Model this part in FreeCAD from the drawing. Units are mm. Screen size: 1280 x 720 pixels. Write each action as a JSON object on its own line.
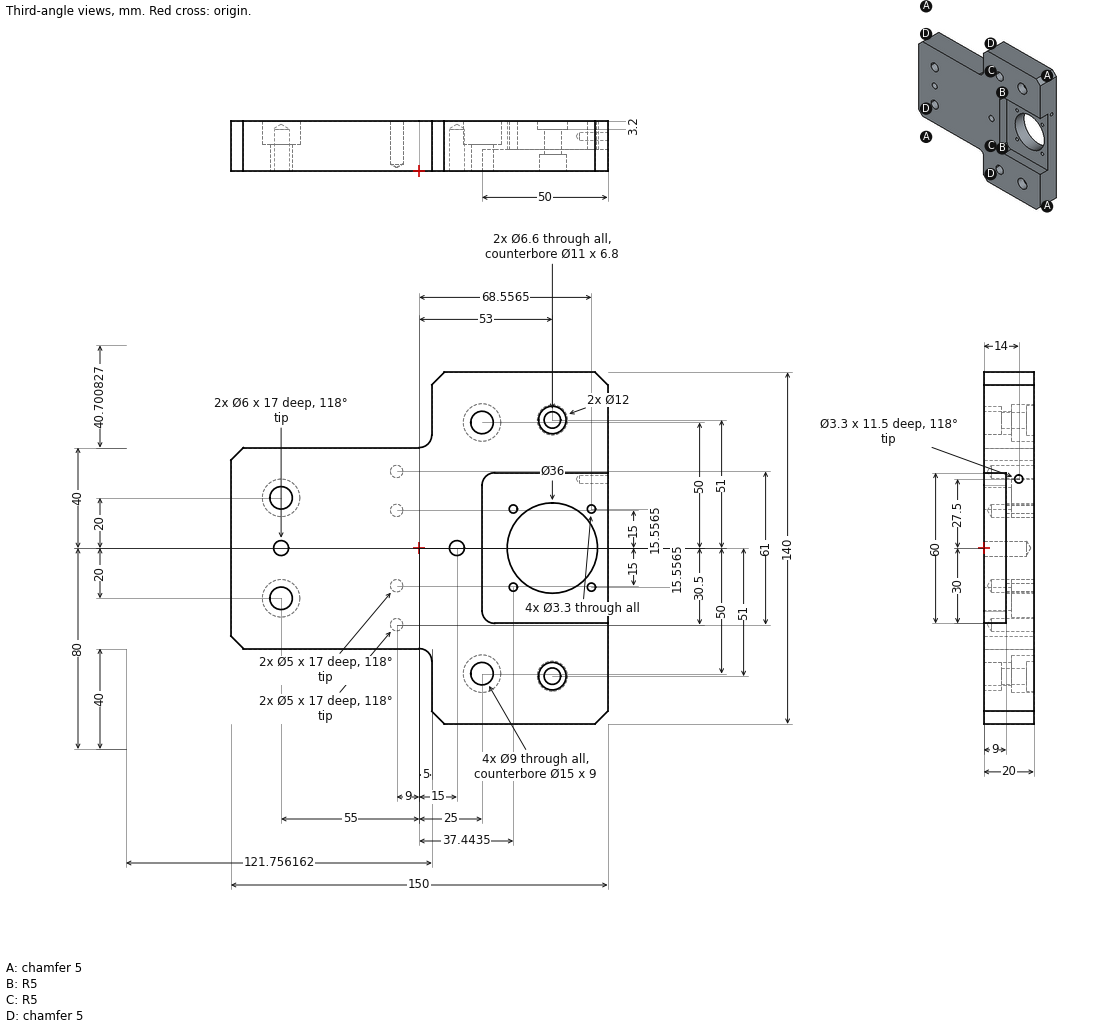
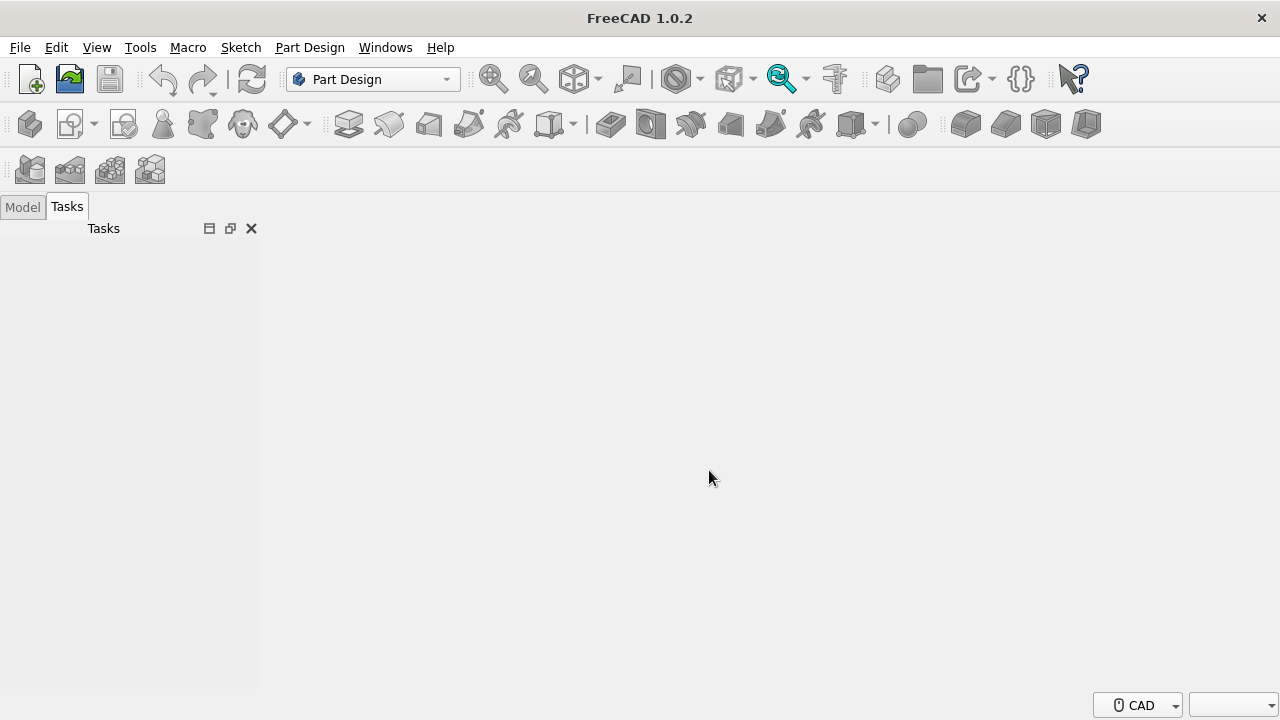
{"action": "left_click", "coordinate": [30, 80]}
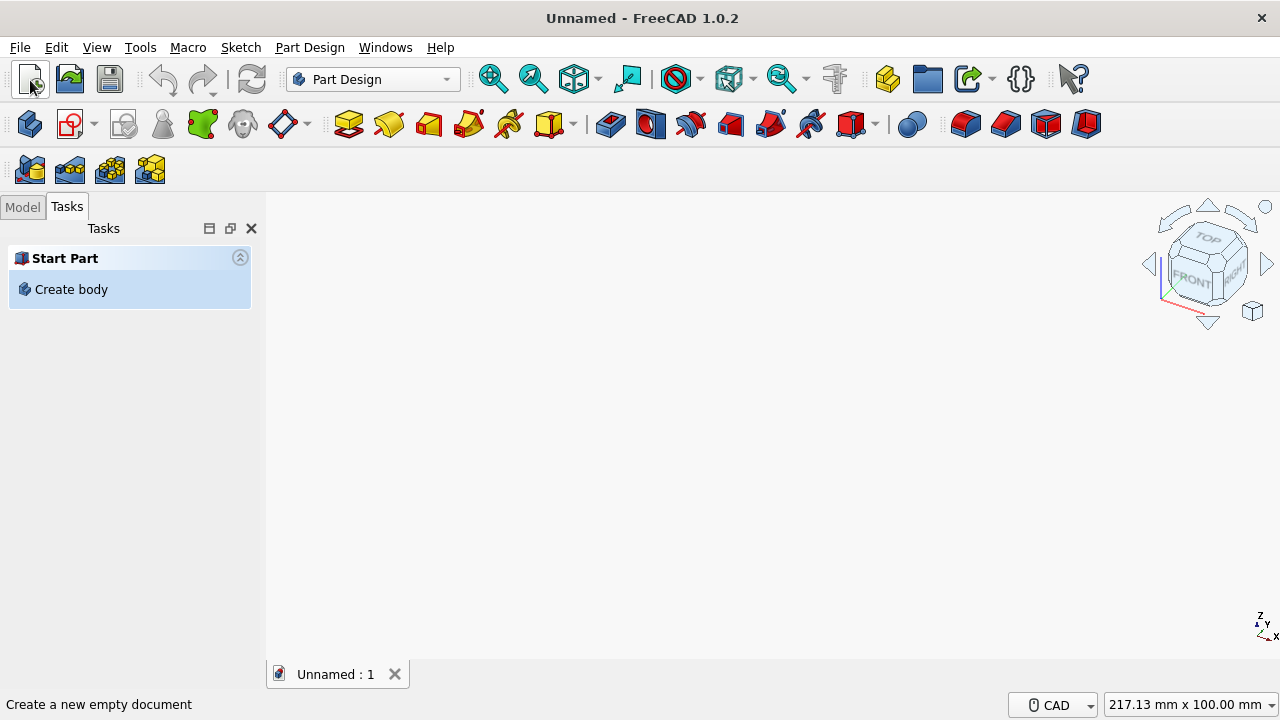
{"action": "left_click", "coordinate": [70, 124]}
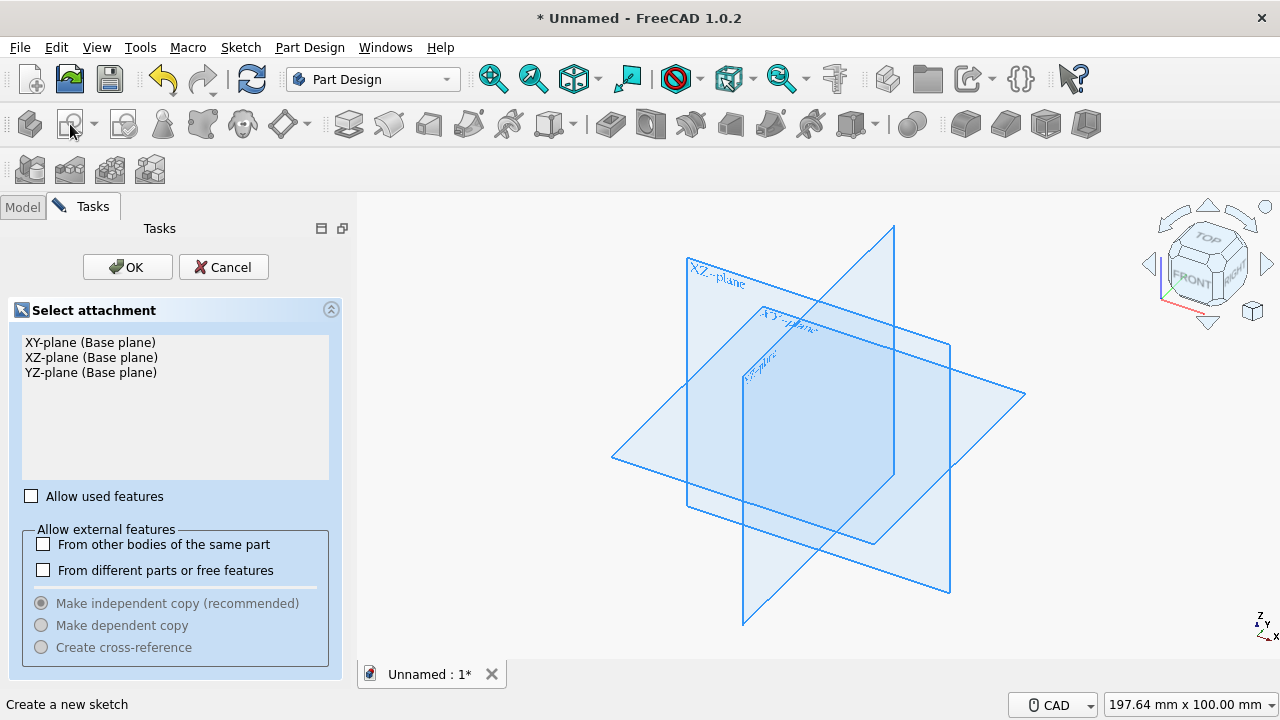
{"action": "left_click", "coordinate": [82, 358]}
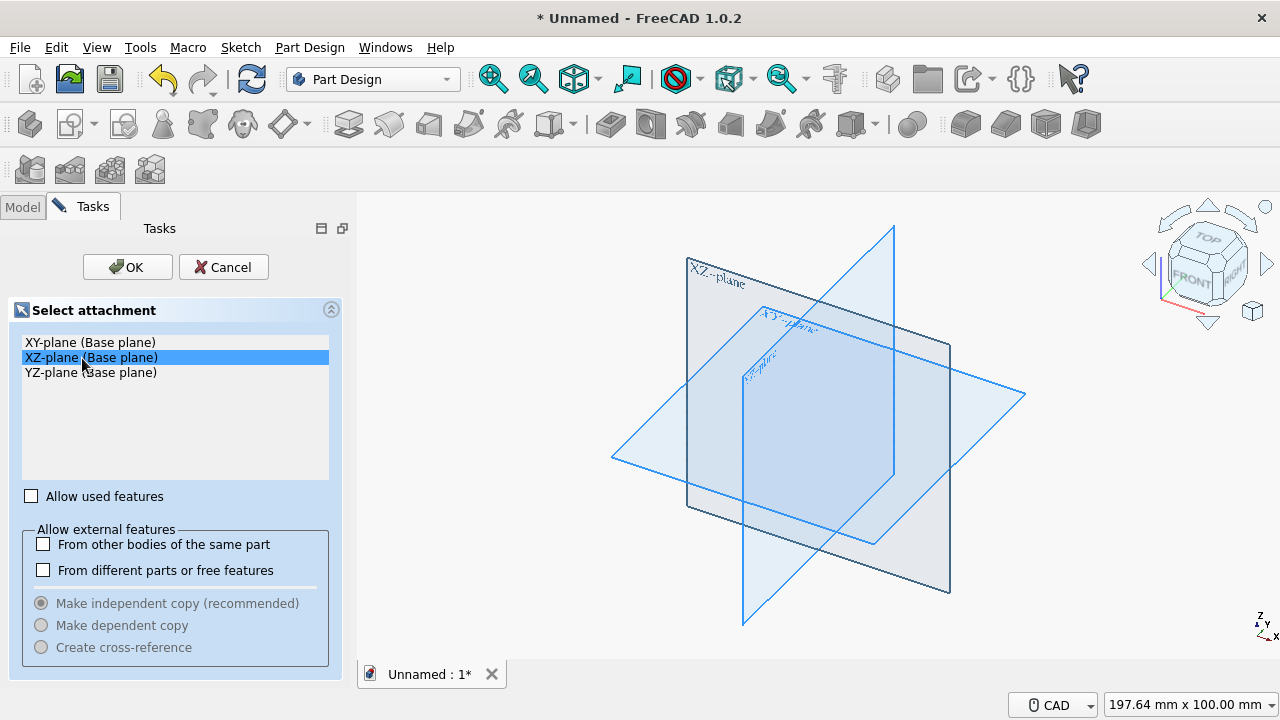
{"action": "left_click", "coordinate": [128, 267]}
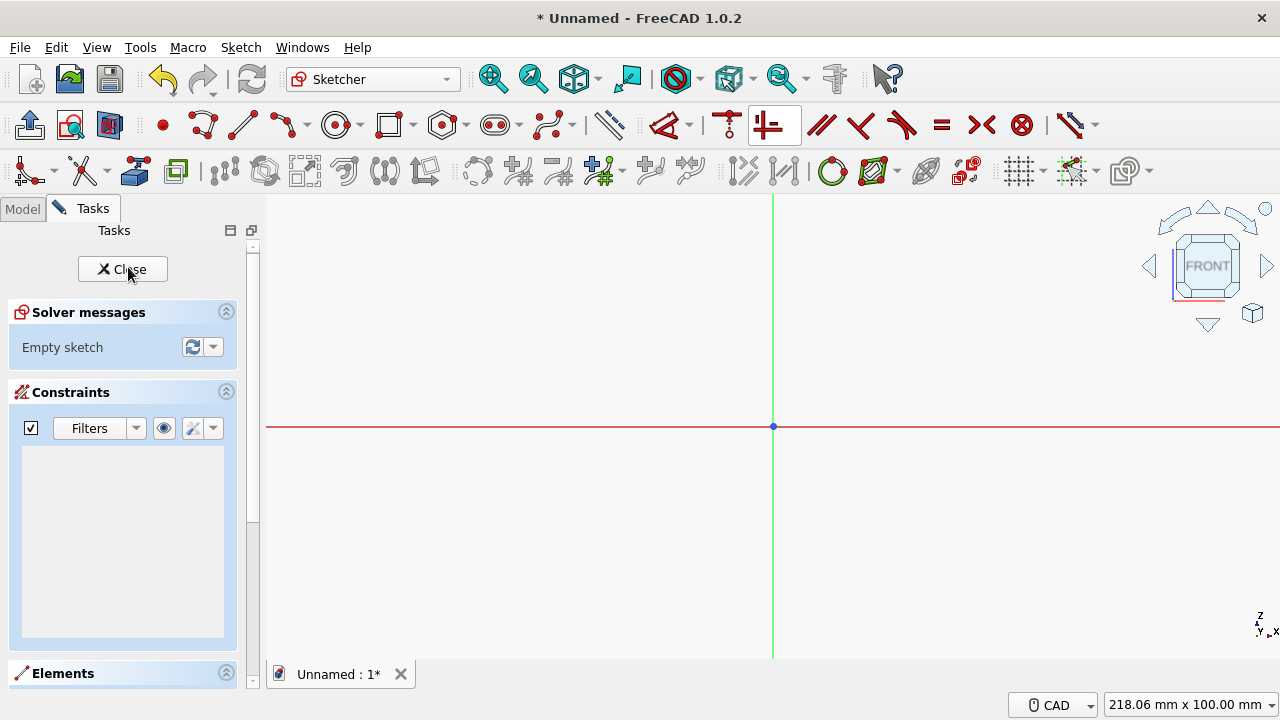
{"action": "scroll", "coordinate": [649, 426], "scroll_direction": "down", "scroll_amount": 4}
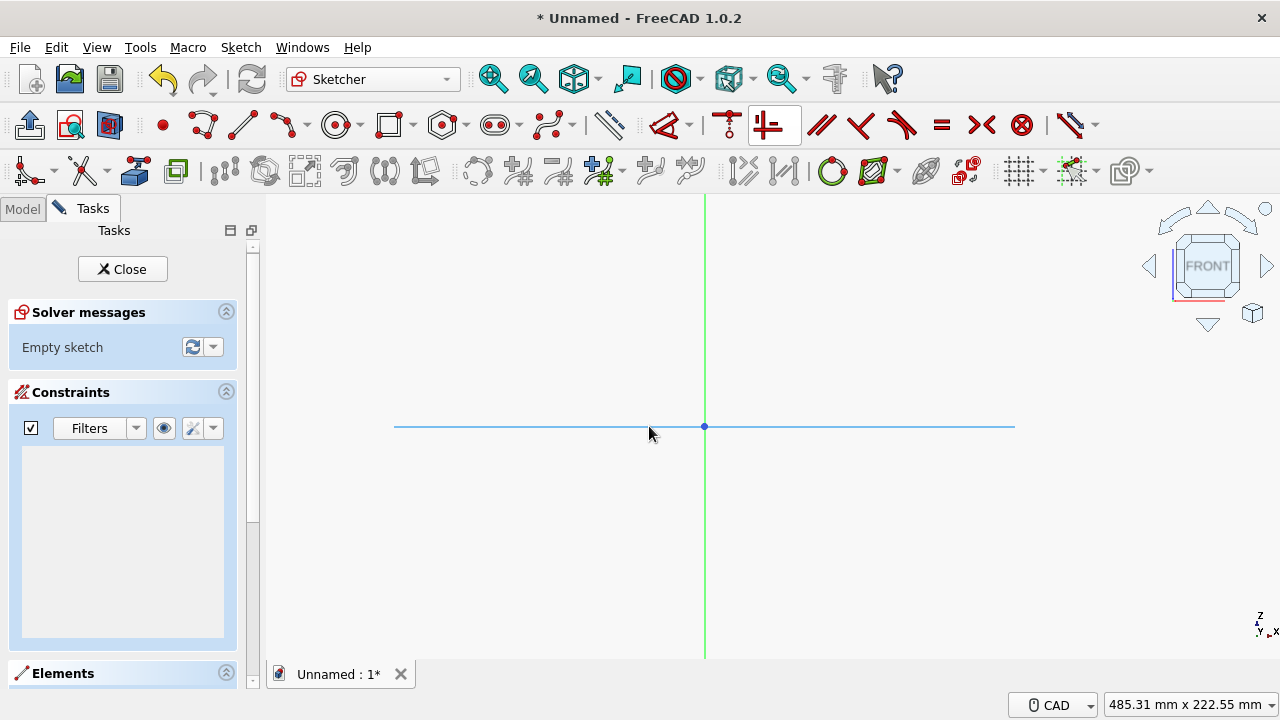
{"action": "left_click", "coordinate": [416, 126]}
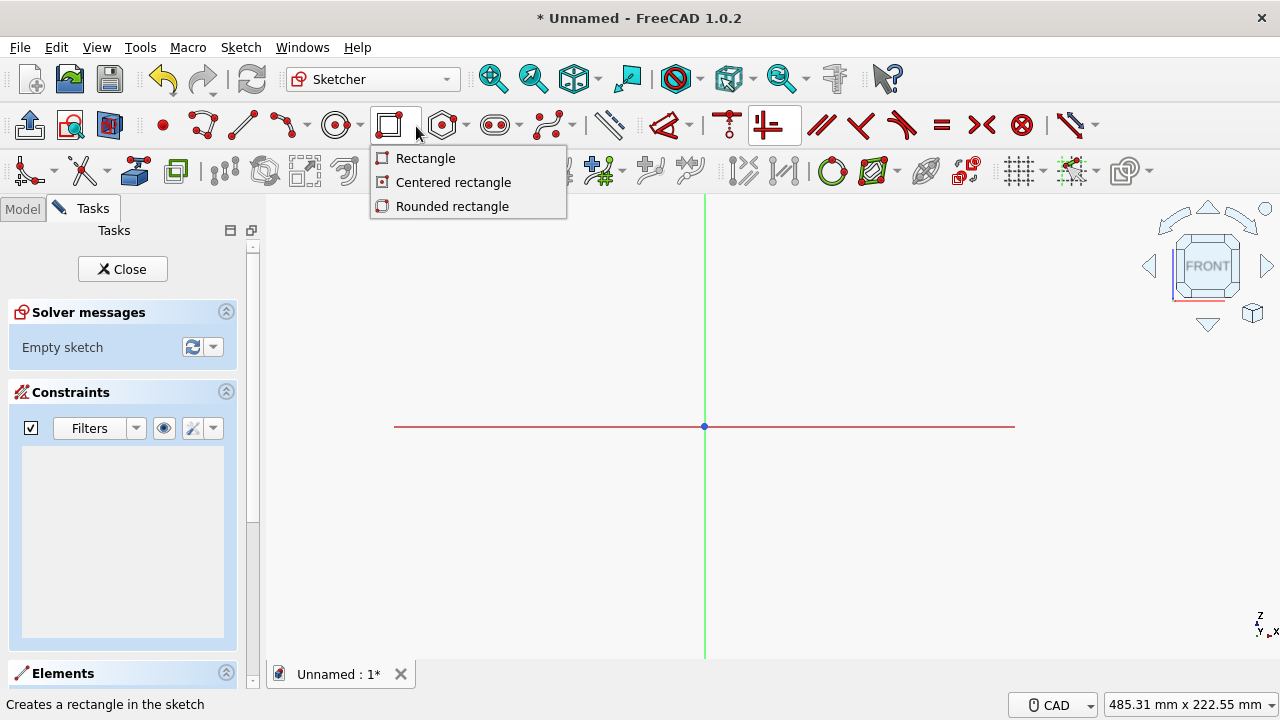
{"action": "left_click", "coordinate": [468, 182]}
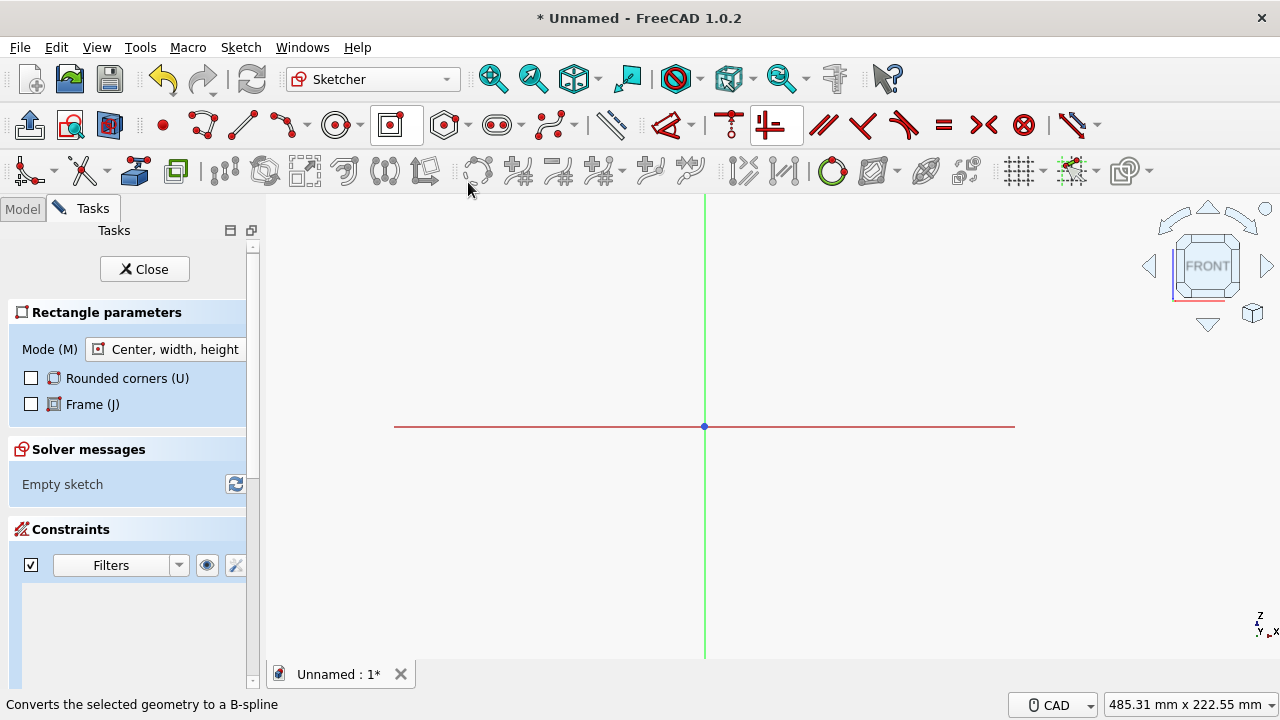
{"action": "left_click", "coordinate": [705, 426]}
{"action": "left_click", "coordinate": [862, 280]}
{"action": "key", "text": "Escape"}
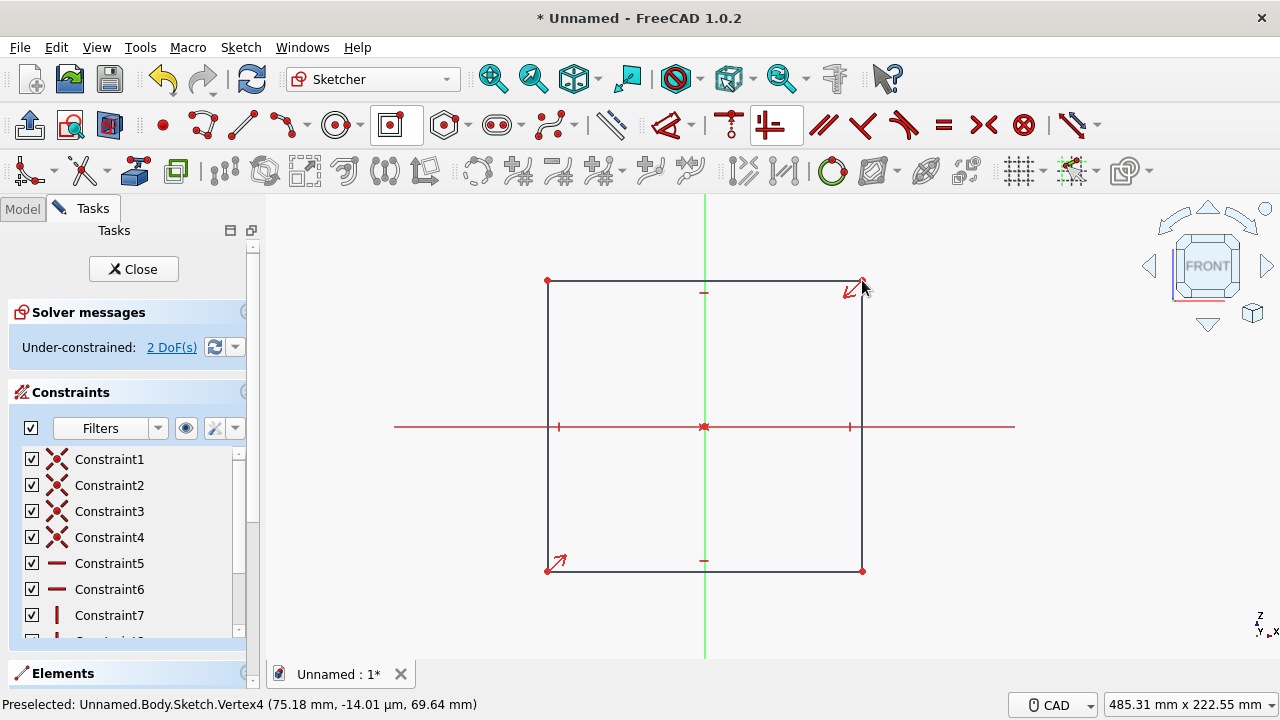
{"action": "left_click", "coordinate": [666, 126]}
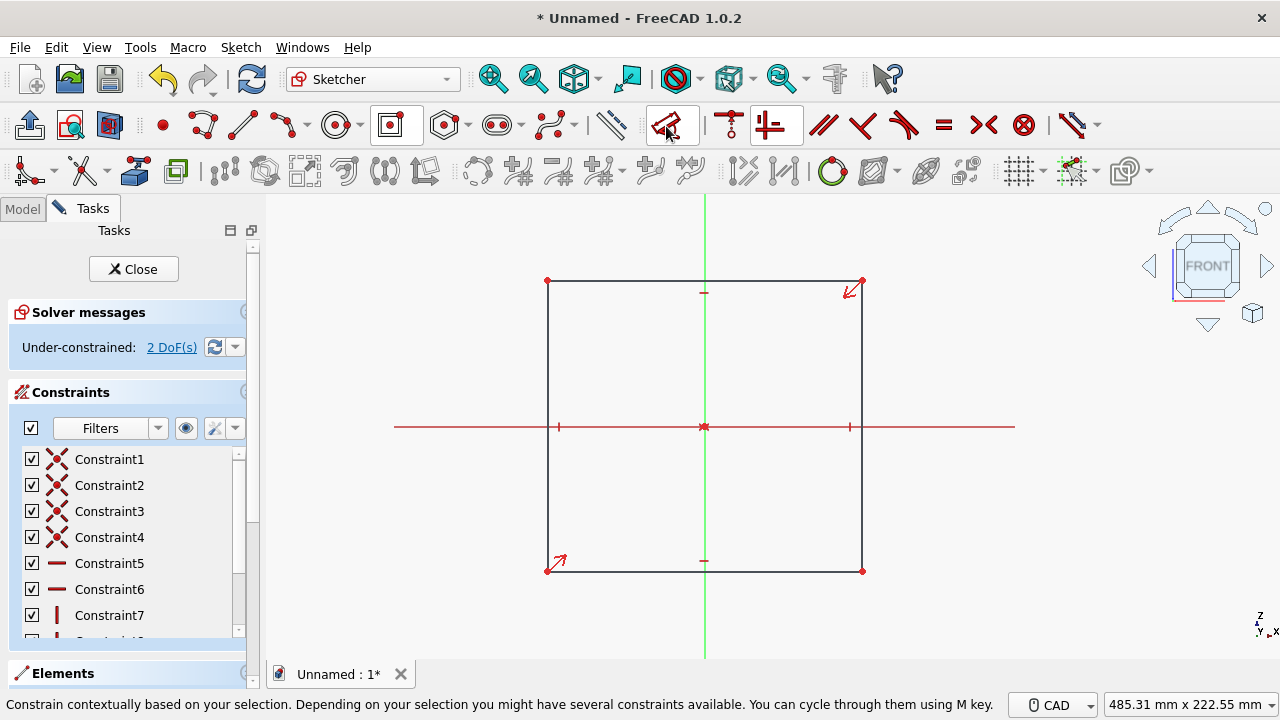
{"action": "left_click", "coordinate": [642, 572]}
{"action": "left_click", "coordinate": [633, 606]}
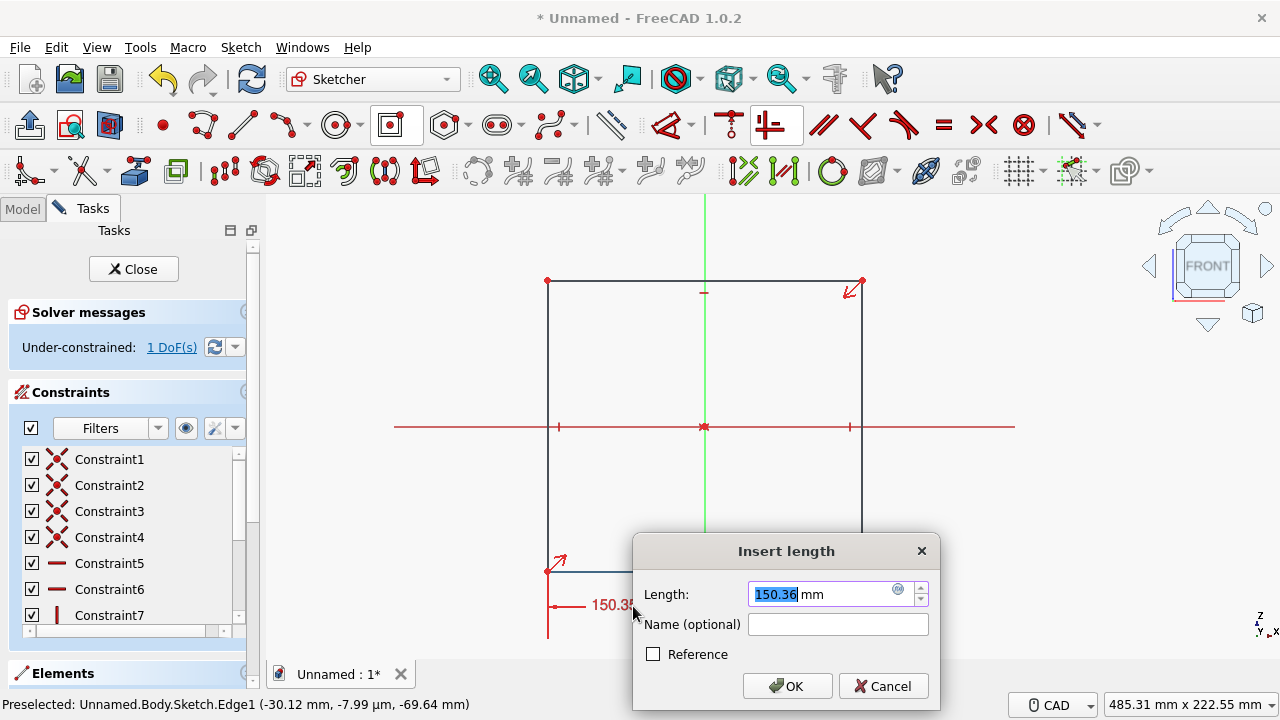
{"action": "type", "text": "150"}
{"action": "key", "text": "Return"}